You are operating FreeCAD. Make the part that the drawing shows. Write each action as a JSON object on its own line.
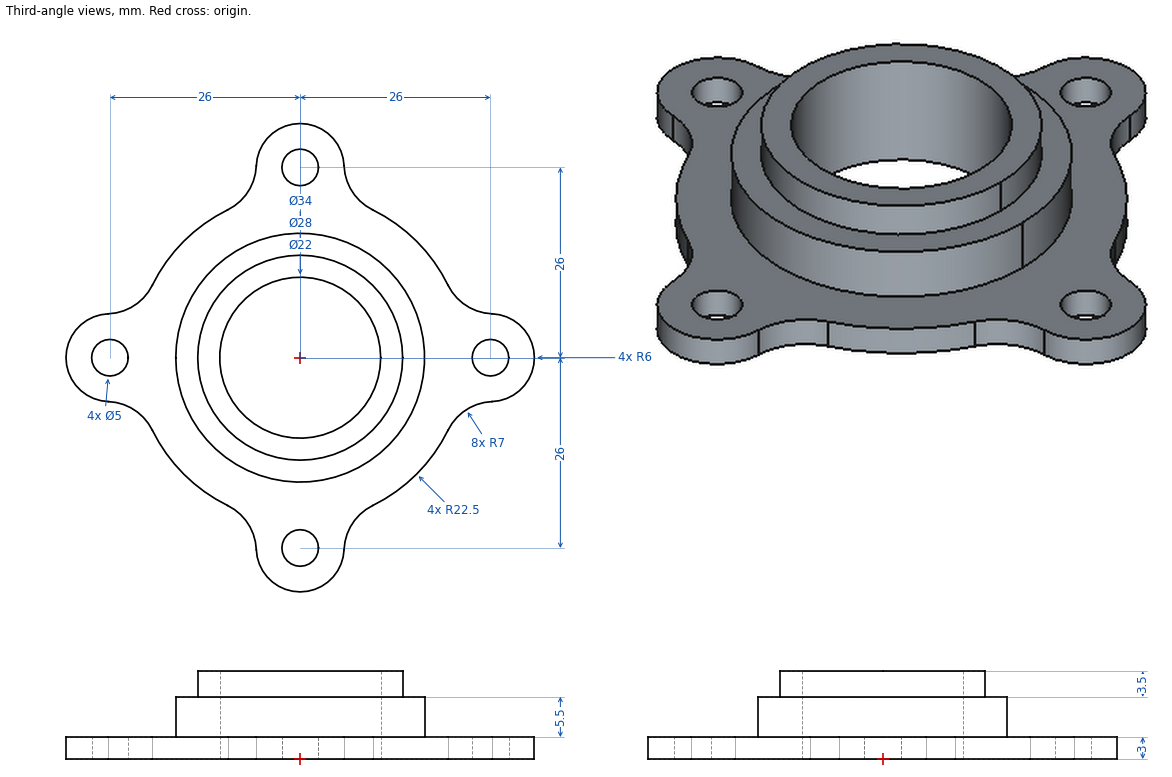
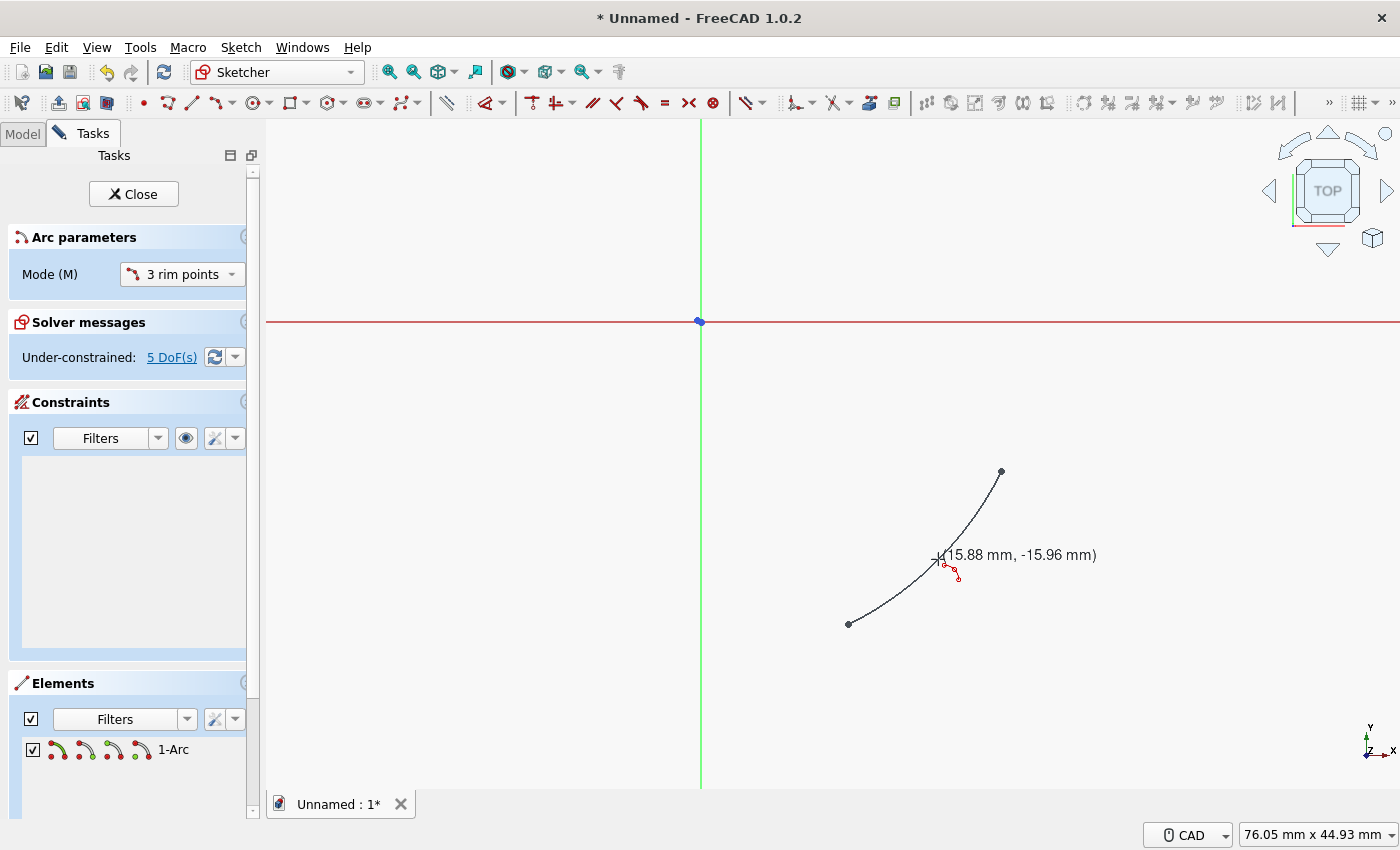
{"action": "left_click", "coordinate": [1002, 471]}
{"action": "left_click", "coordinate": [1092, 411]}
{"action": "left_click", "coordinate": [1039, 428]}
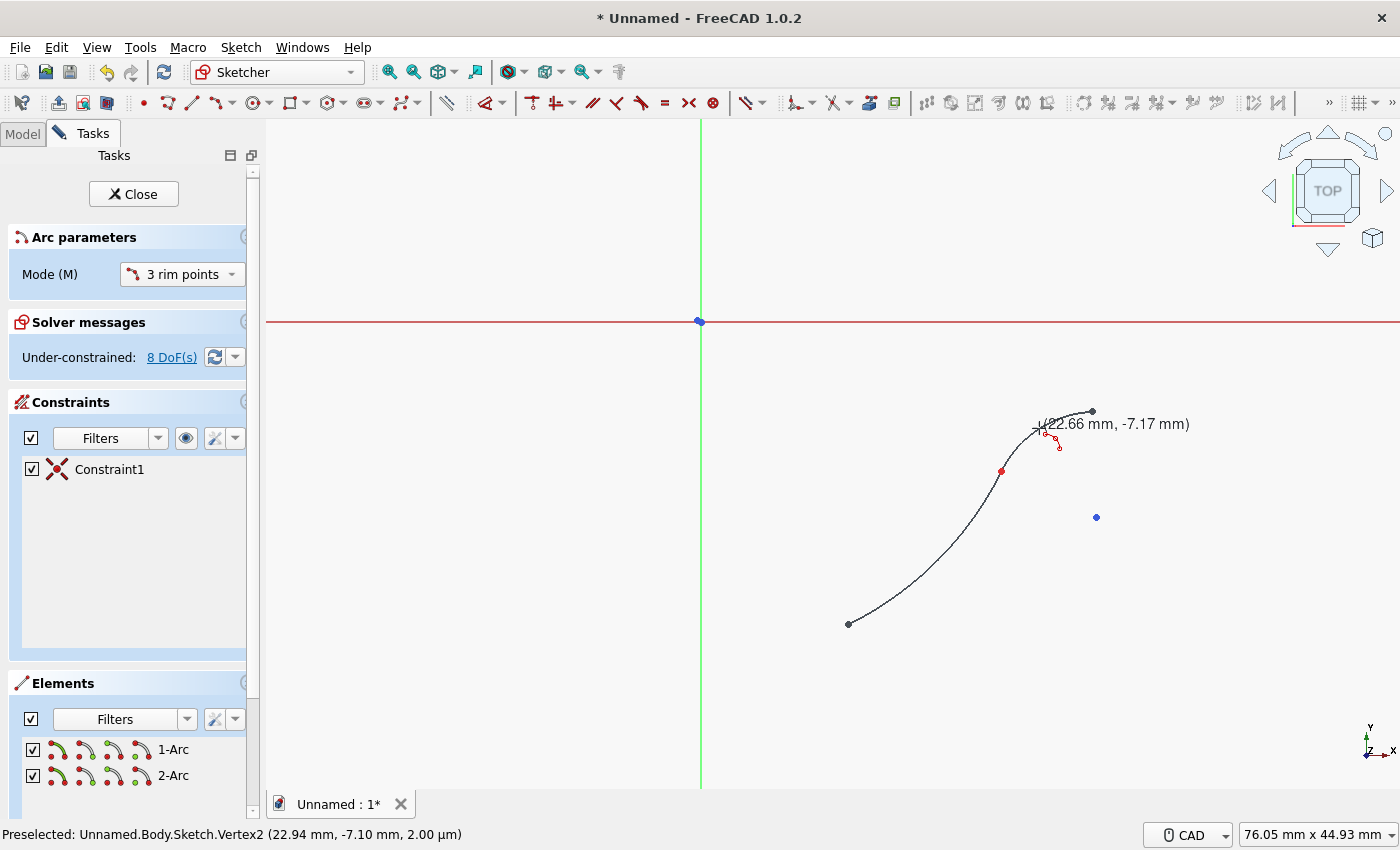
{"action": "left_click", "coordinate": [1092, 412]}
{"action": "left_click", "coordinate": [1092, 233]}
{"action": "left_click", "coordinate": [1162, 374]}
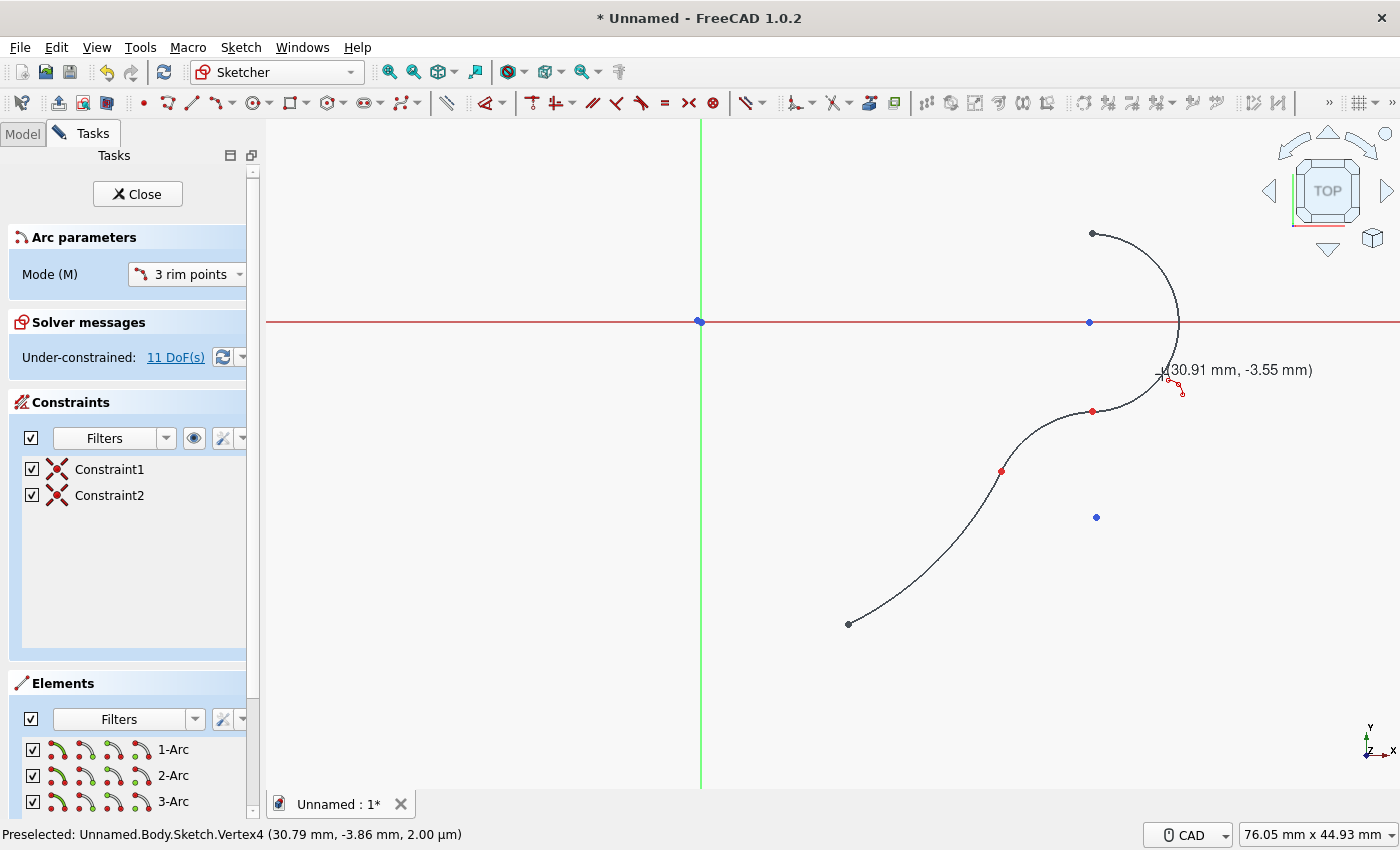
{"action": "left_click", "coordinate": [1092, 234]}
{"action": "left_click", "coordinate": [1002, 174]}
{"action": "left_click", "coordinate": [1039, 216]}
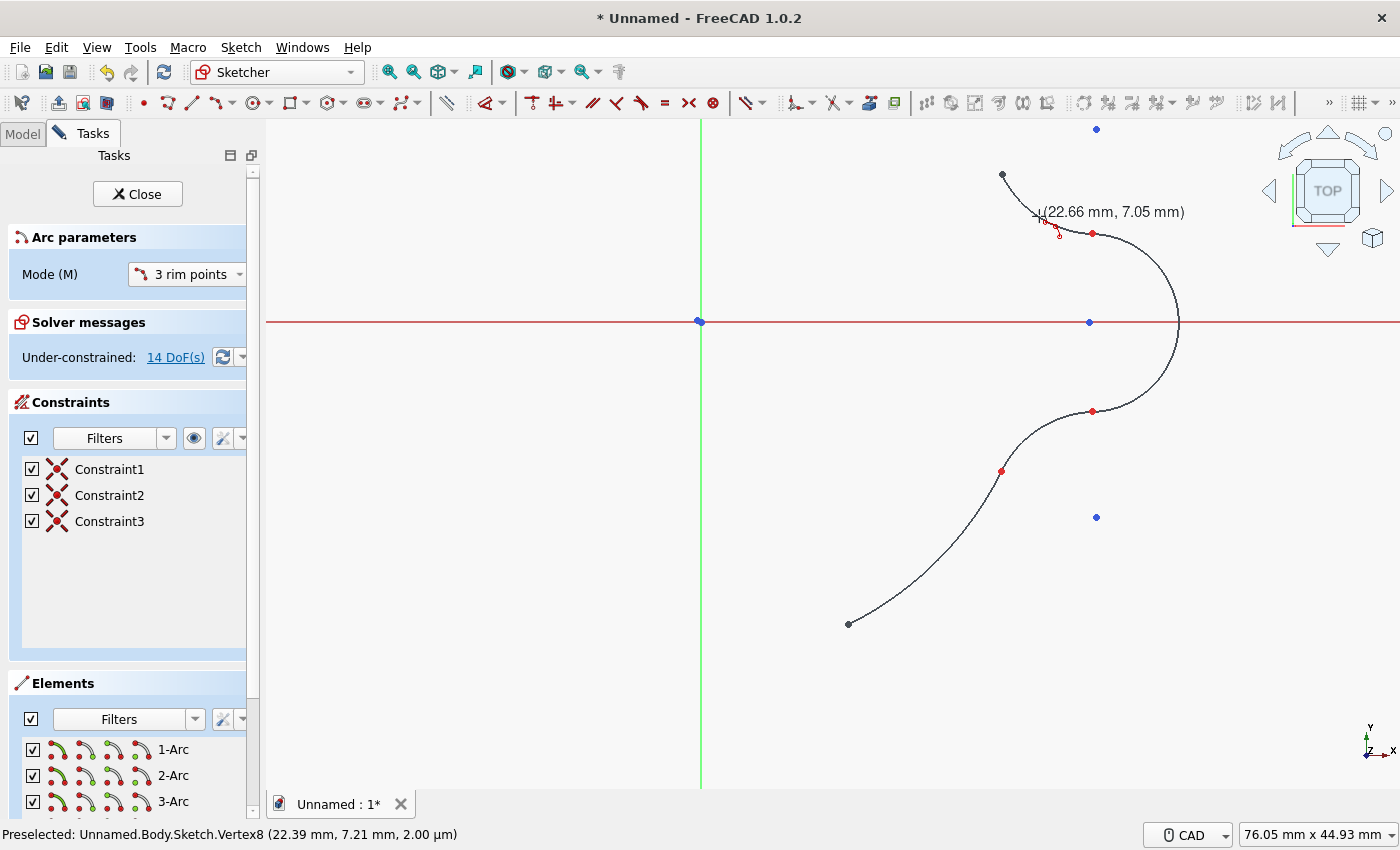
{"action": "left_click", "coordinate": [1002, 175]}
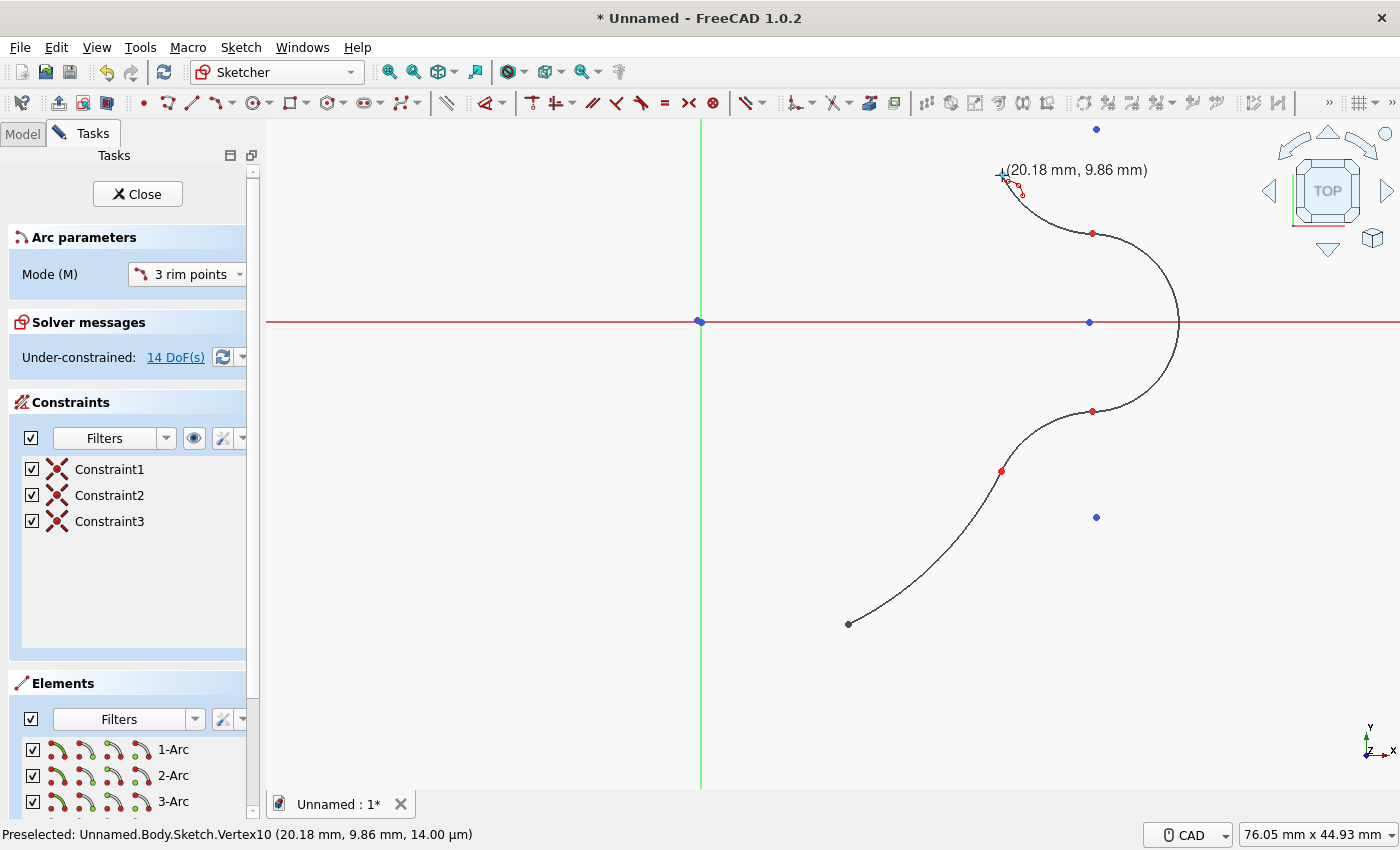
{"action": "scroll", "coordinate": [816, 562], "scroll_direction": "down", "scroll_amount": 4}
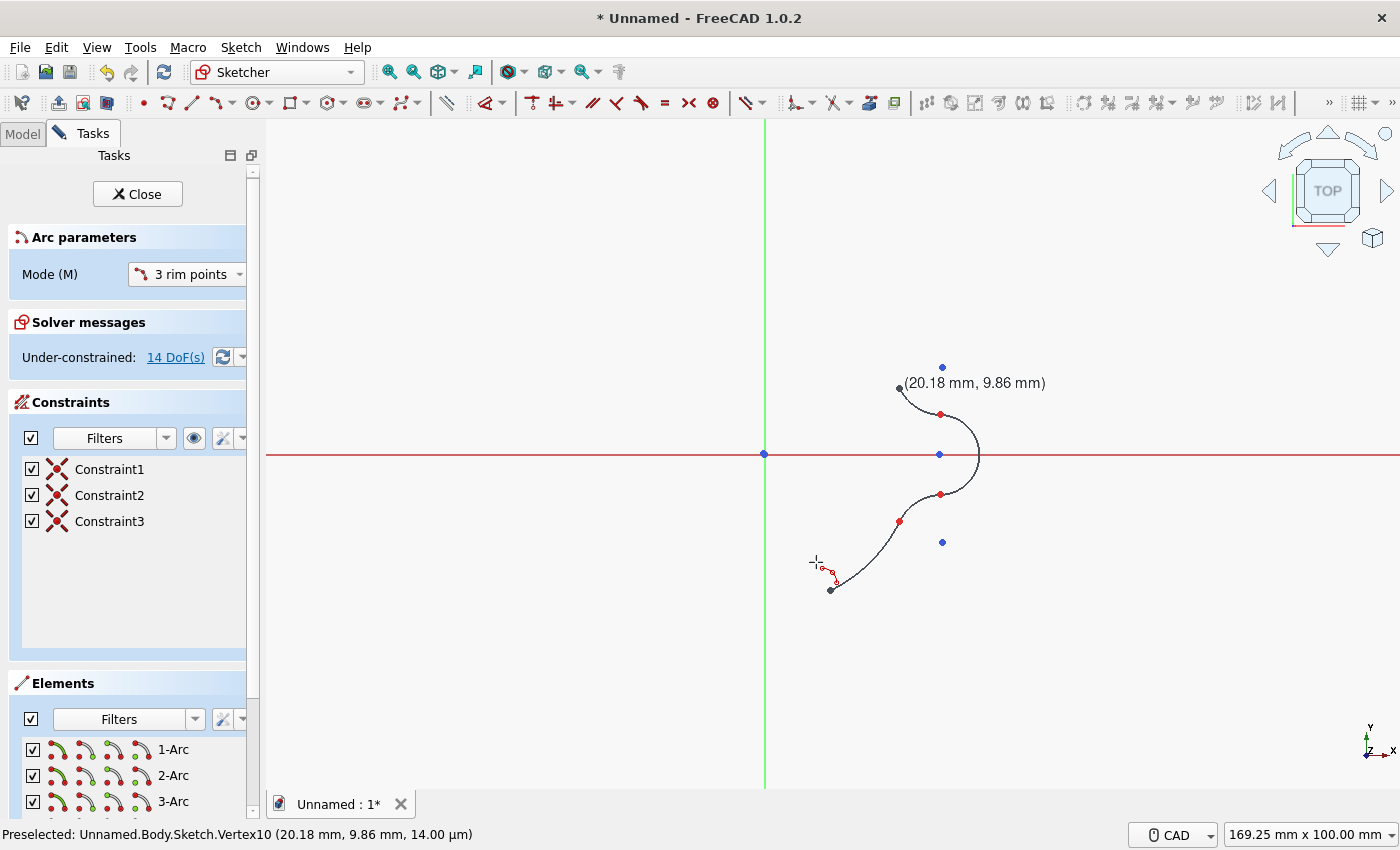
{"action": "left_click", "coordinate": [831, 319]}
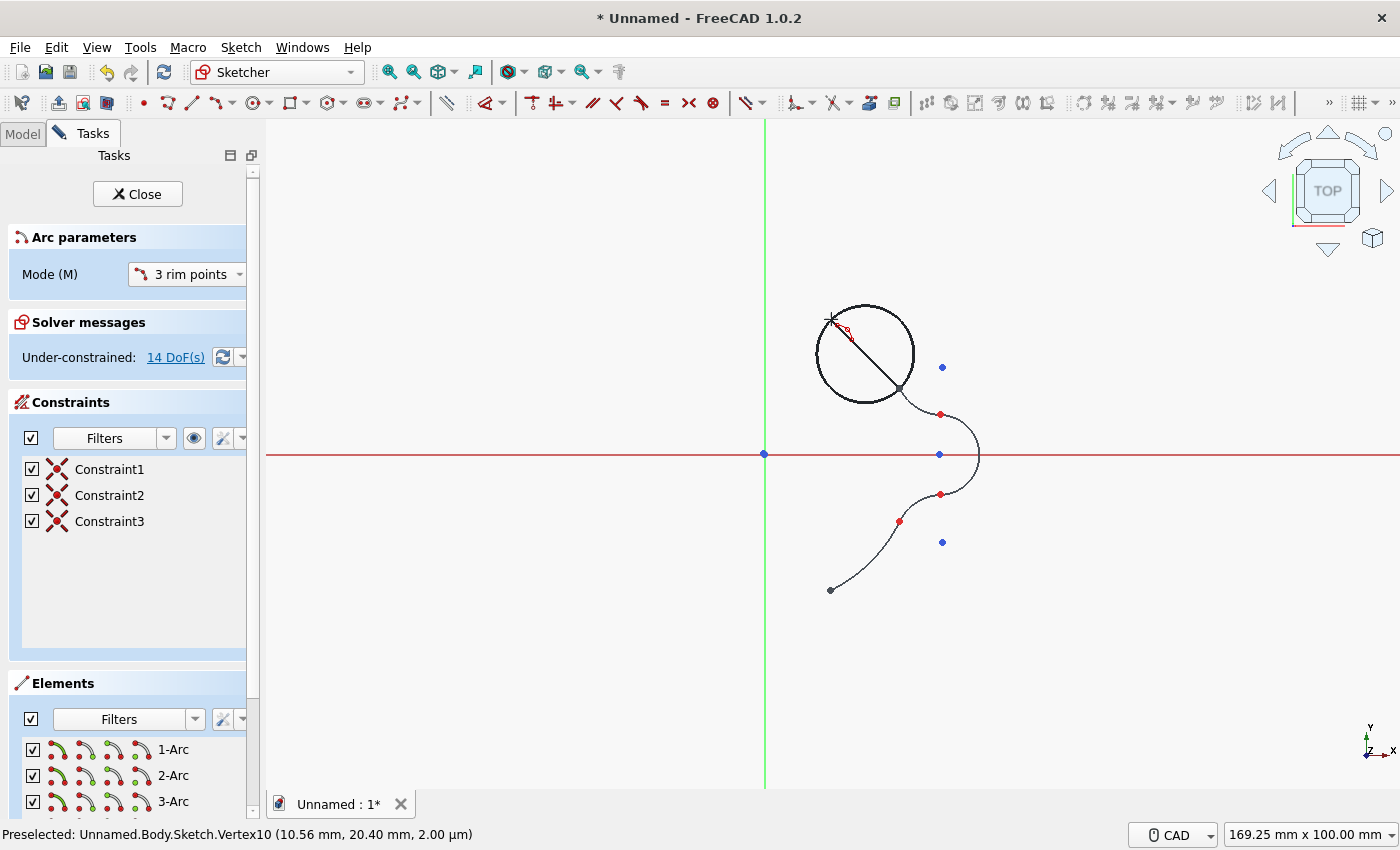
{"action": "scroll", "coordinate": [871, 348], "scroll_direction": "up", "scroll_amount": 4}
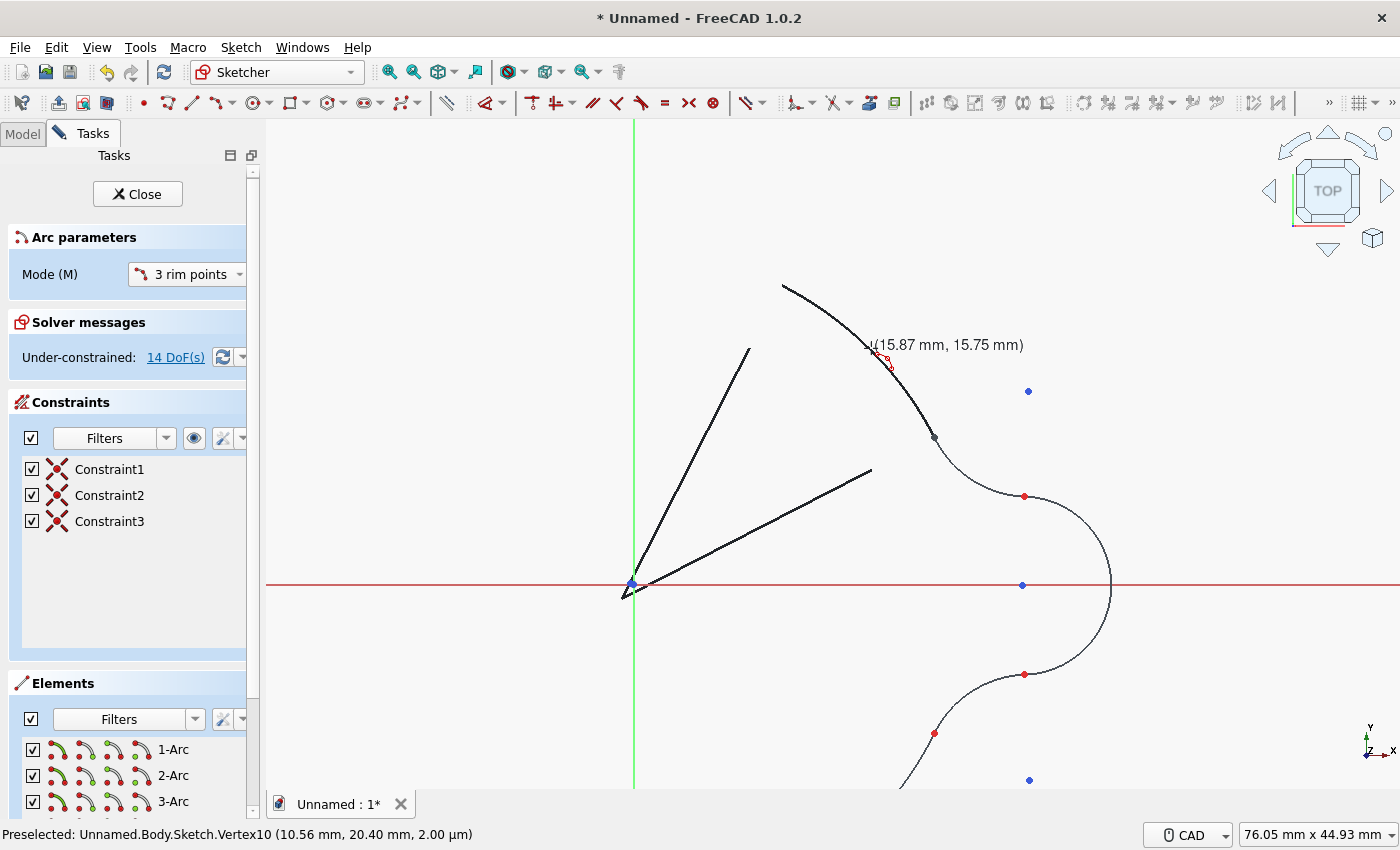
{"action": "left_click", "coordinate": [871, 347]}